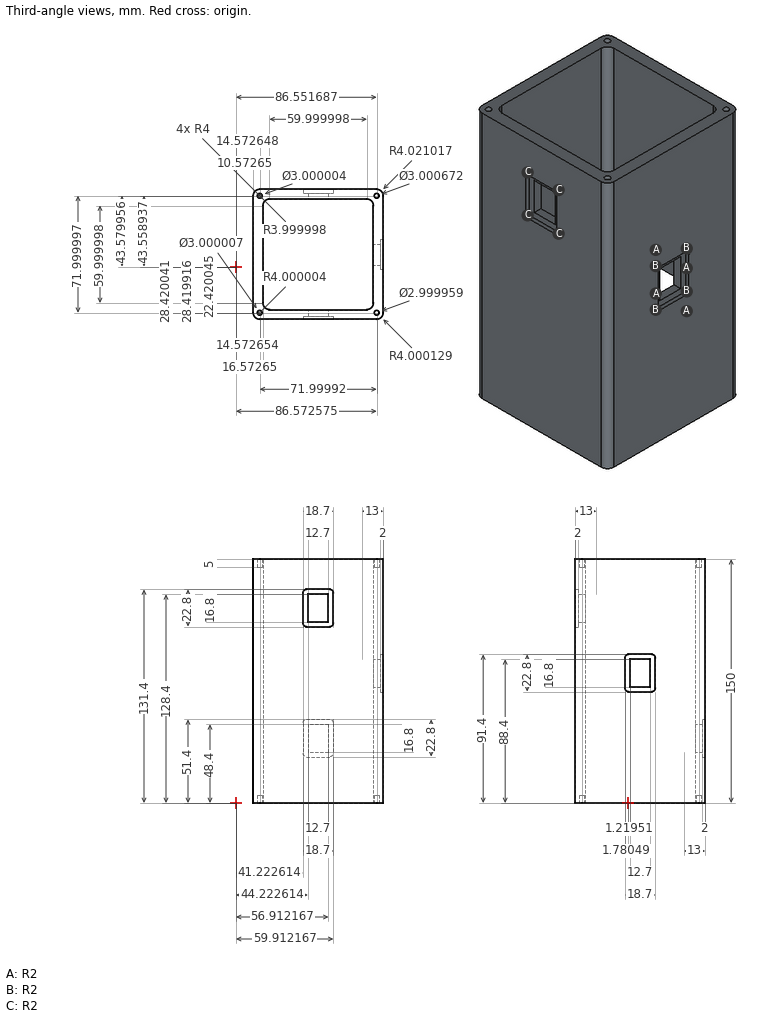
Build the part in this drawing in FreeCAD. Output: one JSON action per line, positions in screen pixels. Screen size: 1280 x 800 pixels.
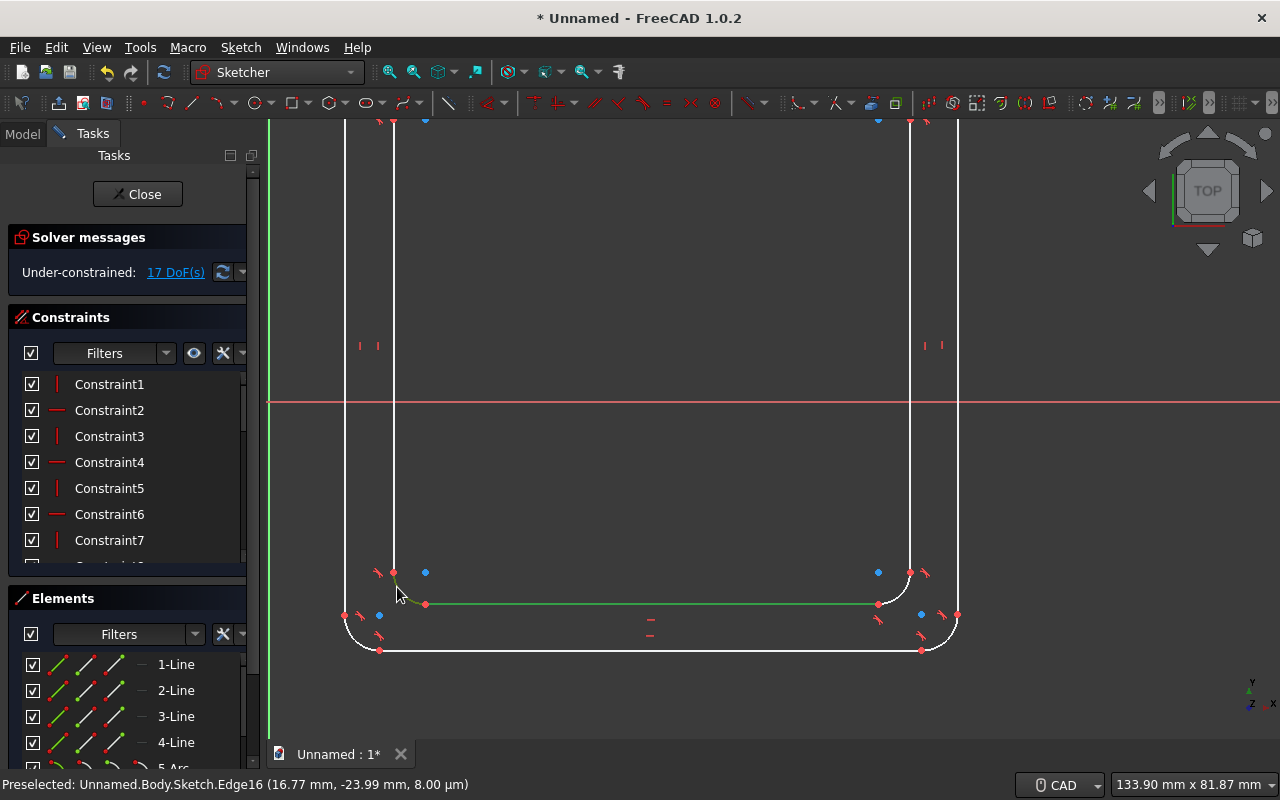
{"action": "left_click", "coordinate": [644, 104]}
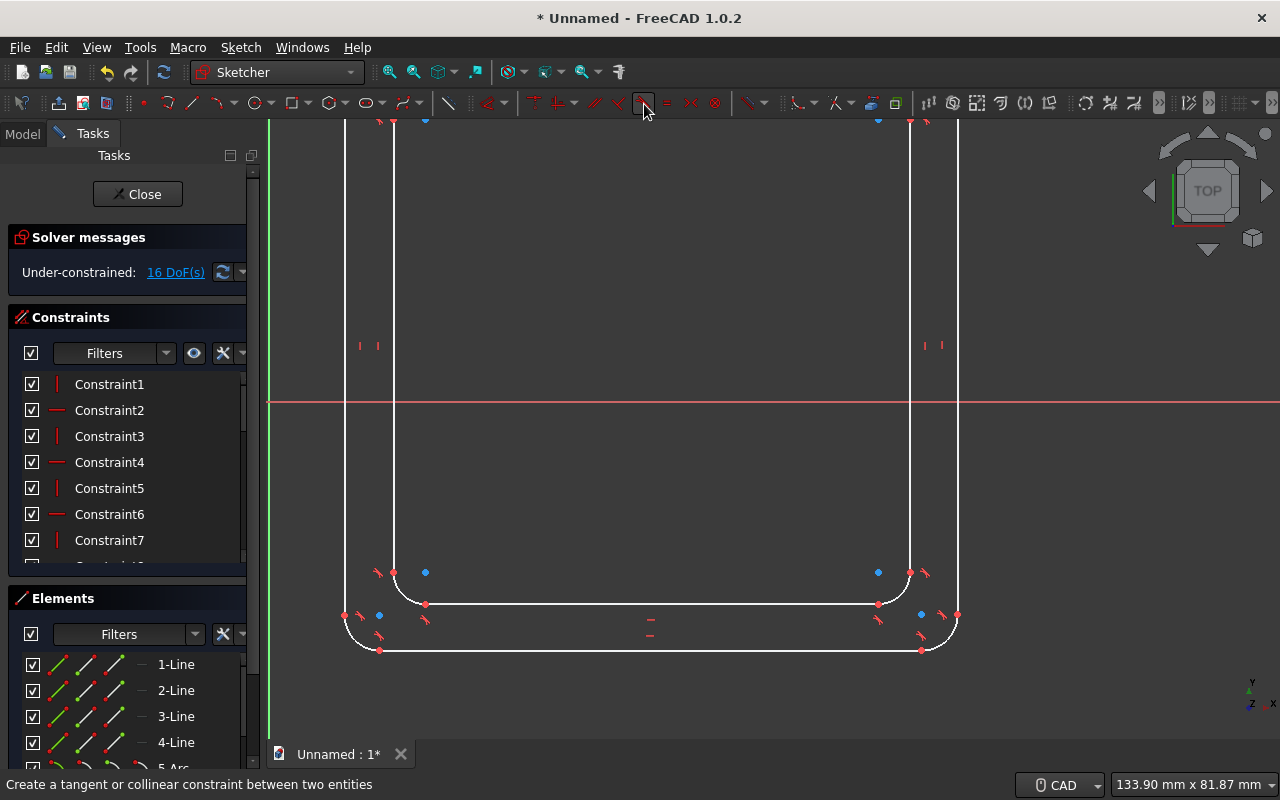
{"action": "scroll", "coordinate": [893, 601], "scroll_direction": "down", "scroll_amount": 2}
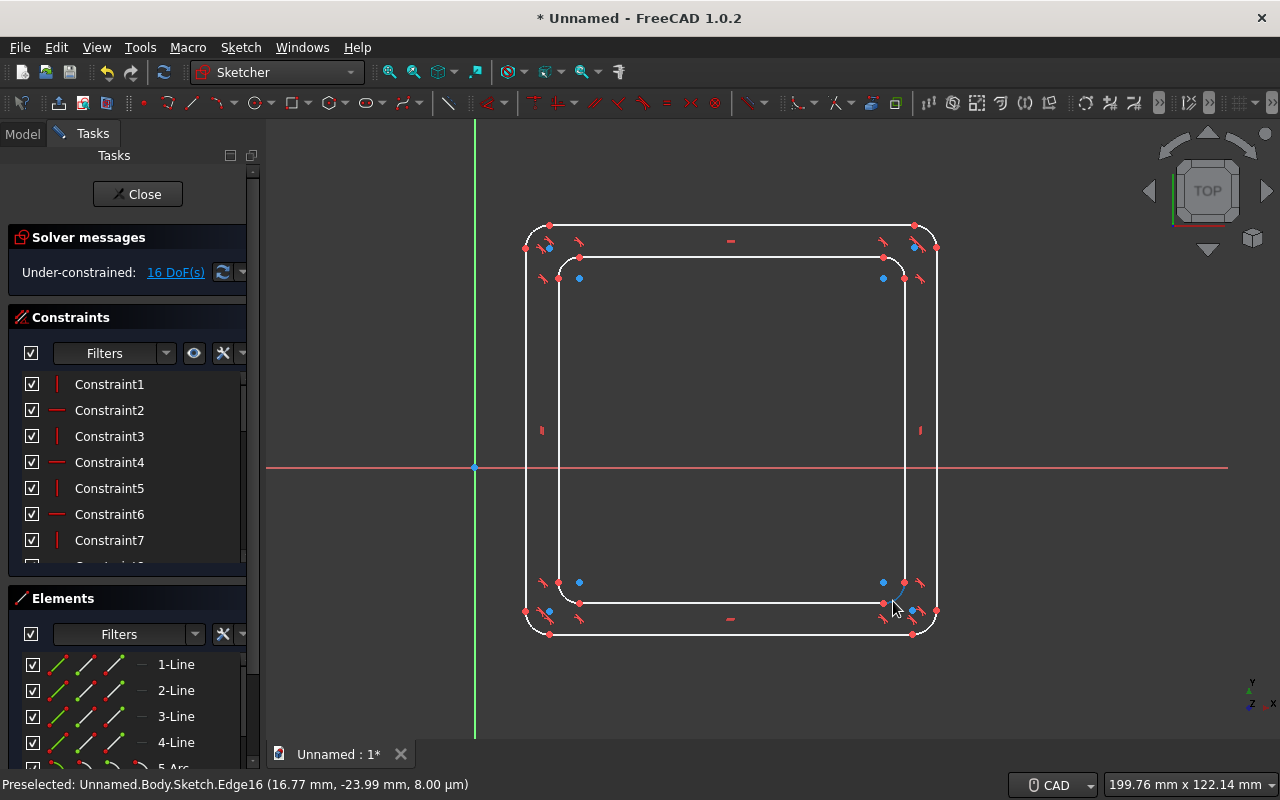
{"action": "scroll", "coordinate": [570, 260], "scroll_direction": "up", "scroll_amount": 2}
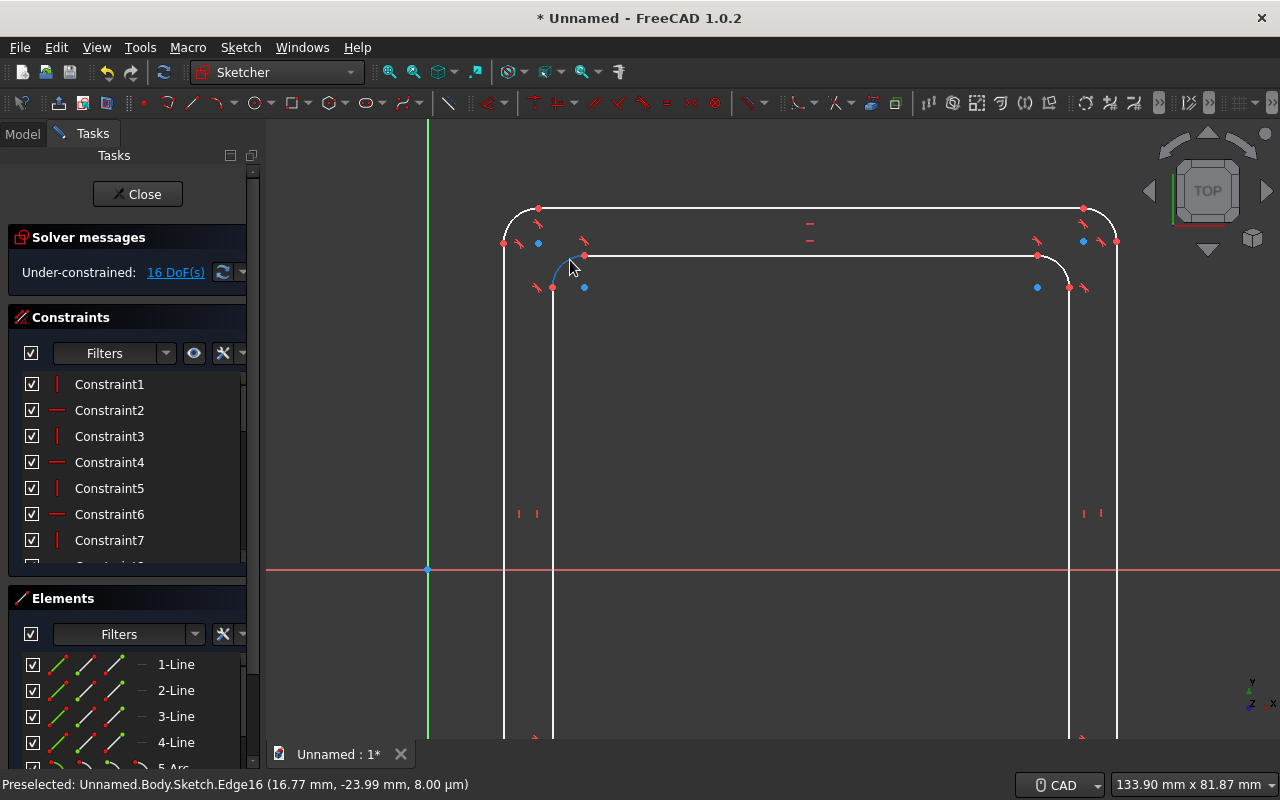
{"action": "left_click", "coordinate": [570, 259]}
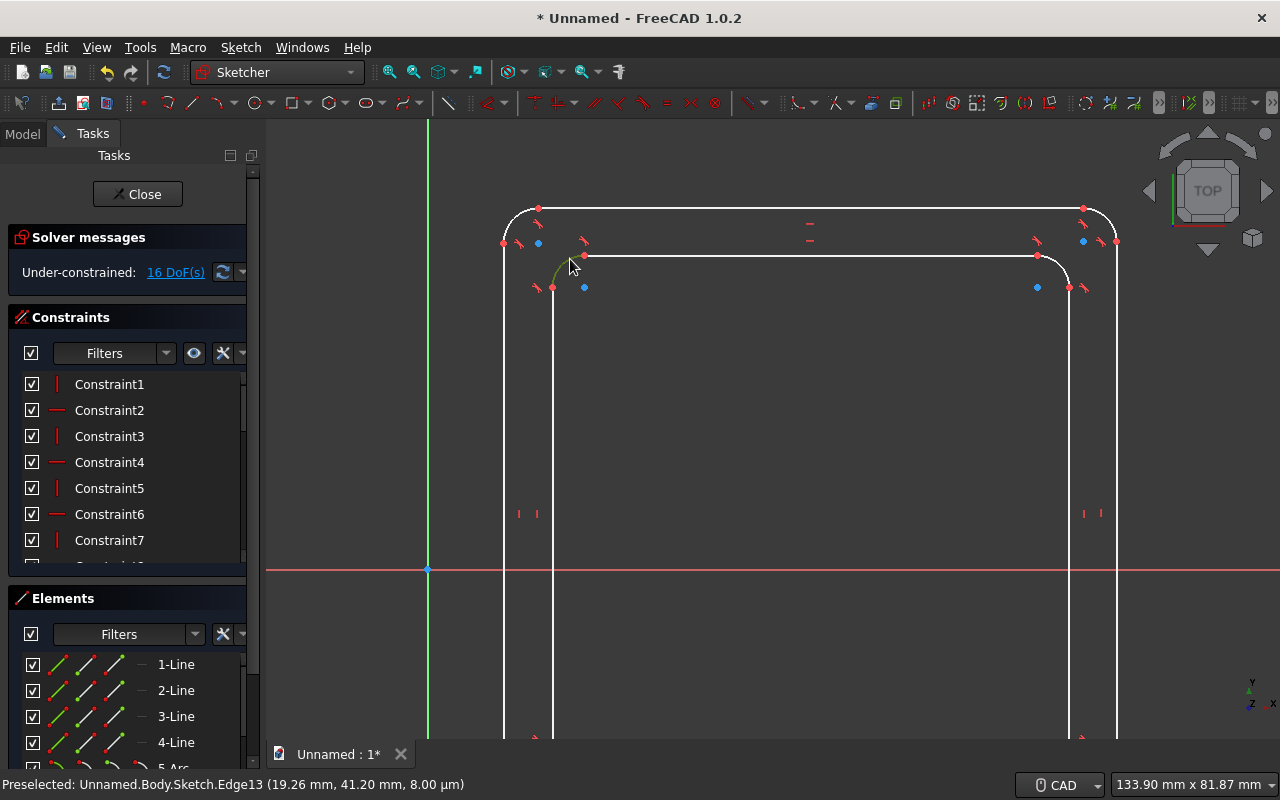
{"action": "left_click", "coordinate": [1066, 273]}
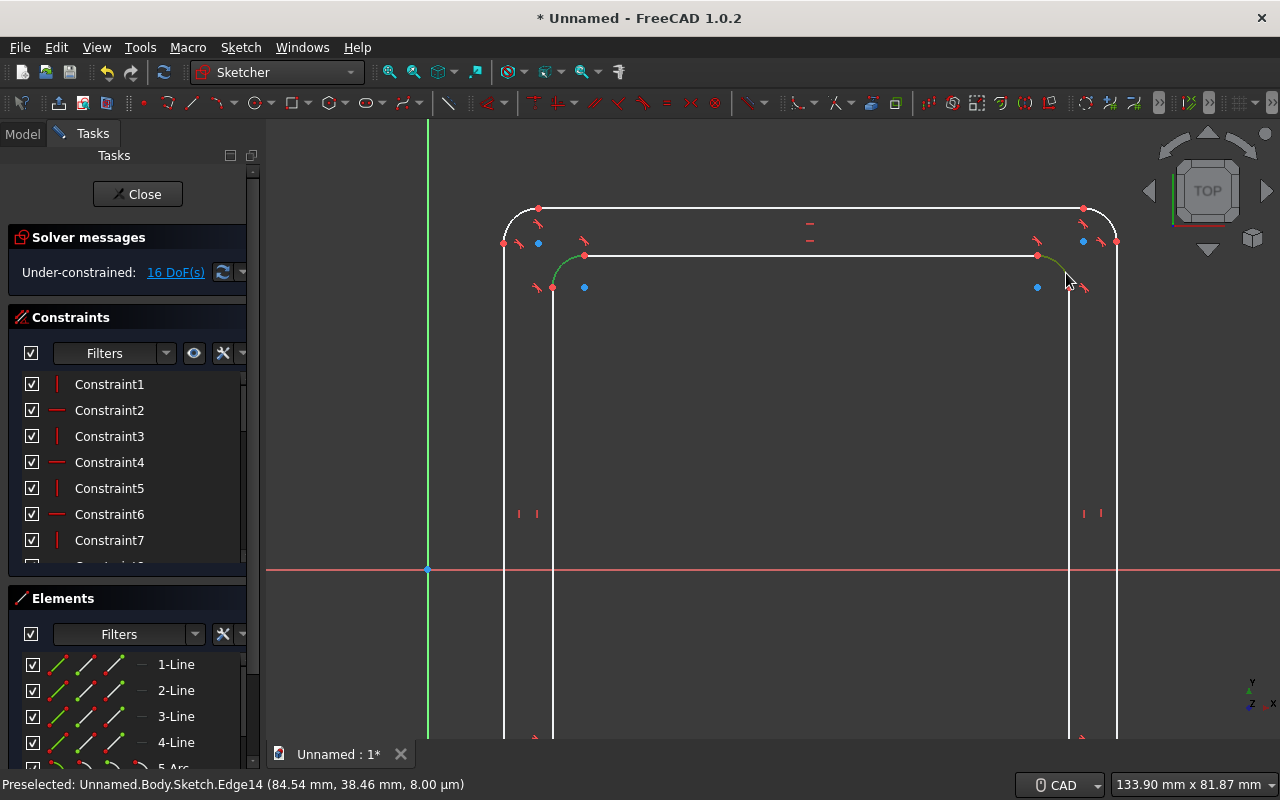
{"action": "scroll", "coordinate": [570, 260], "scroll_direction": "down", "scroll_amount": 2}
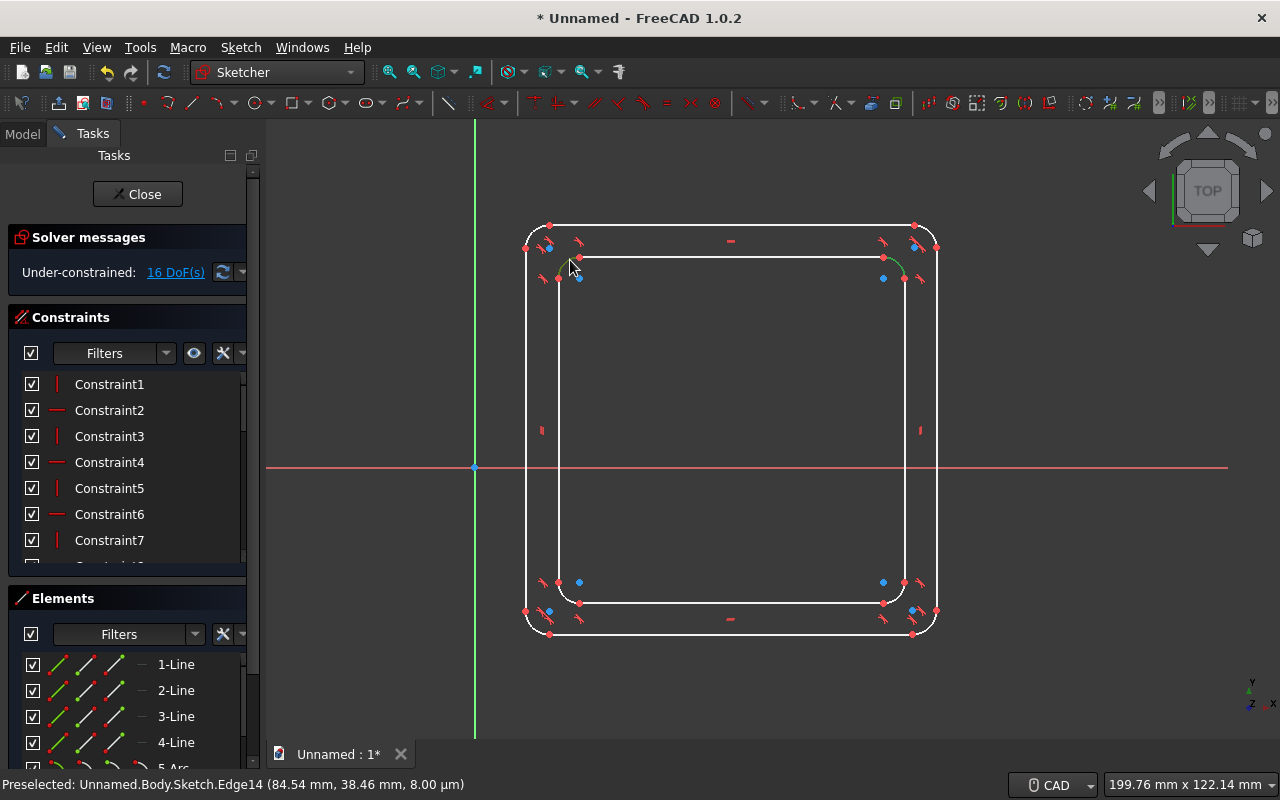
{"action": "scroll", "coordinate": [893, 601], "scroll_direction": "up", "scroll_amount": 2}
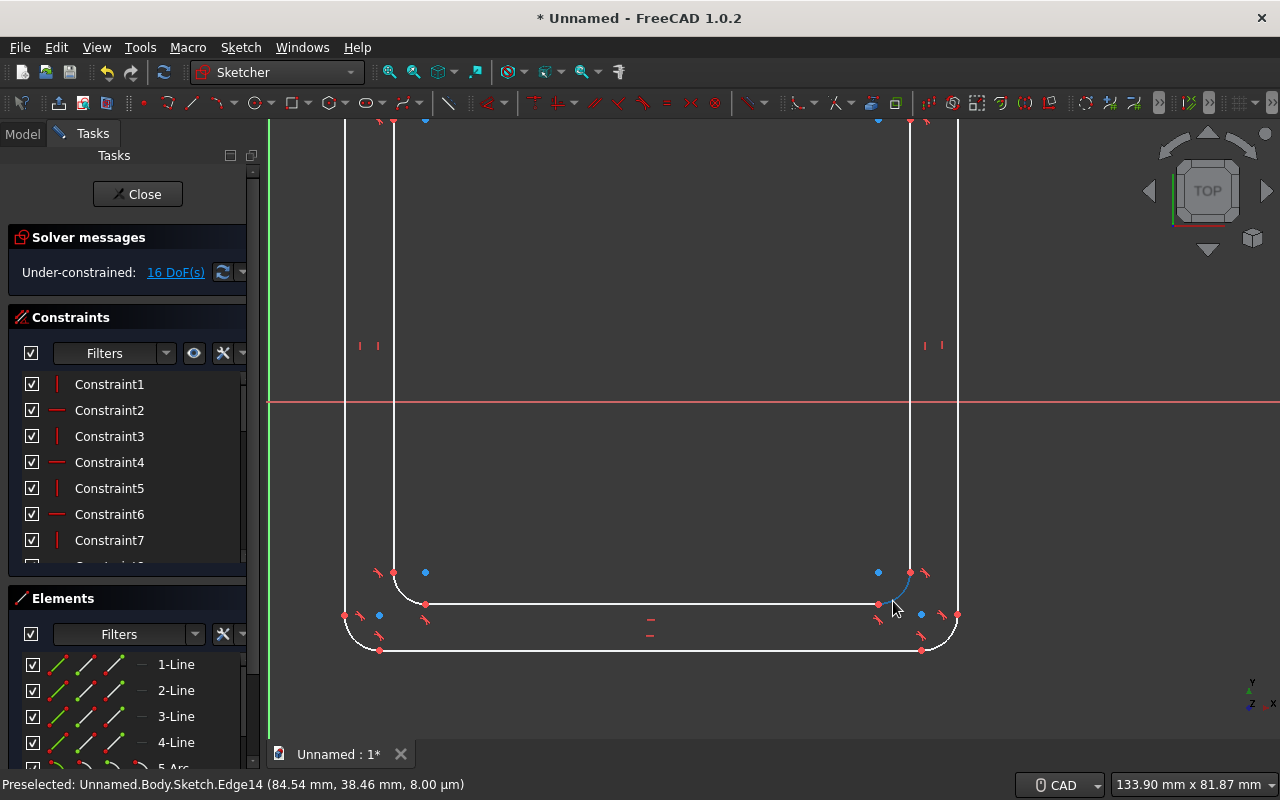
{"action": "left_click", "coordinate": [893, 601]}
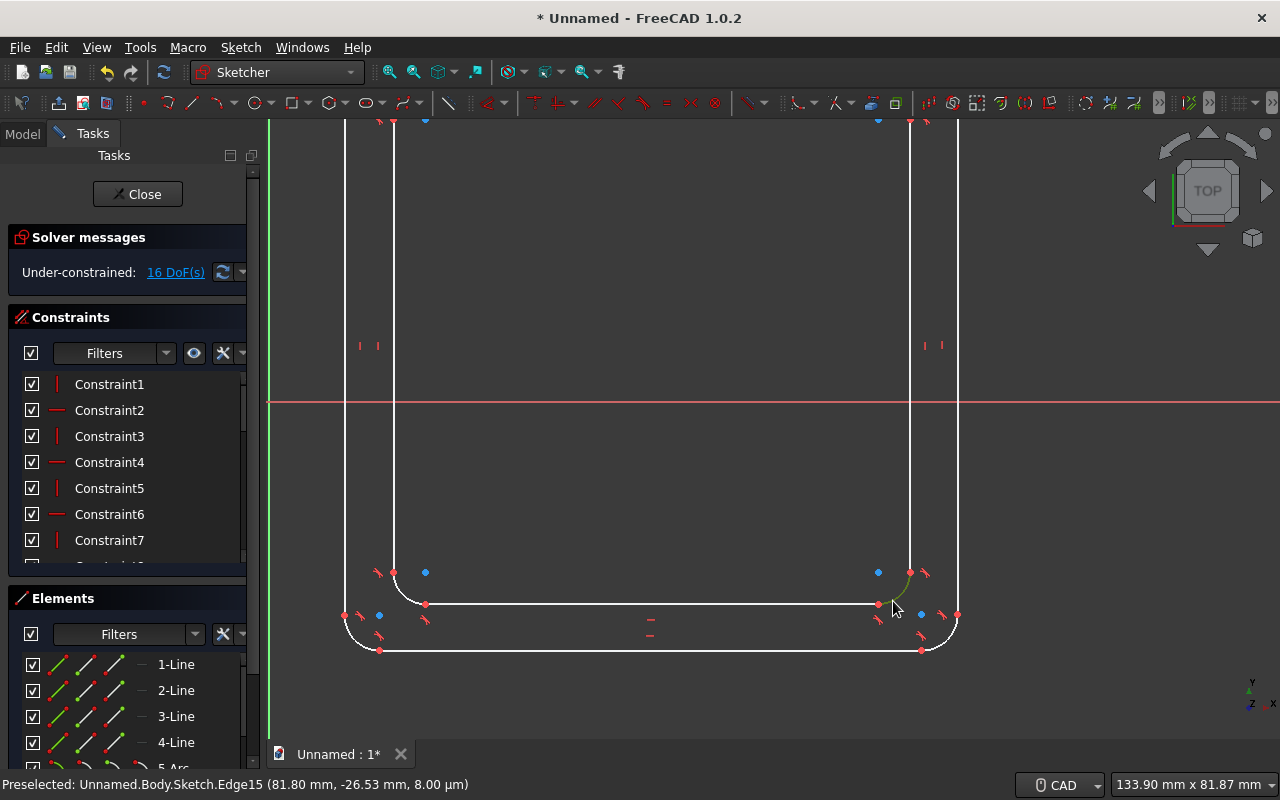
{"action": "left_click", "coordinate": [397, 587]}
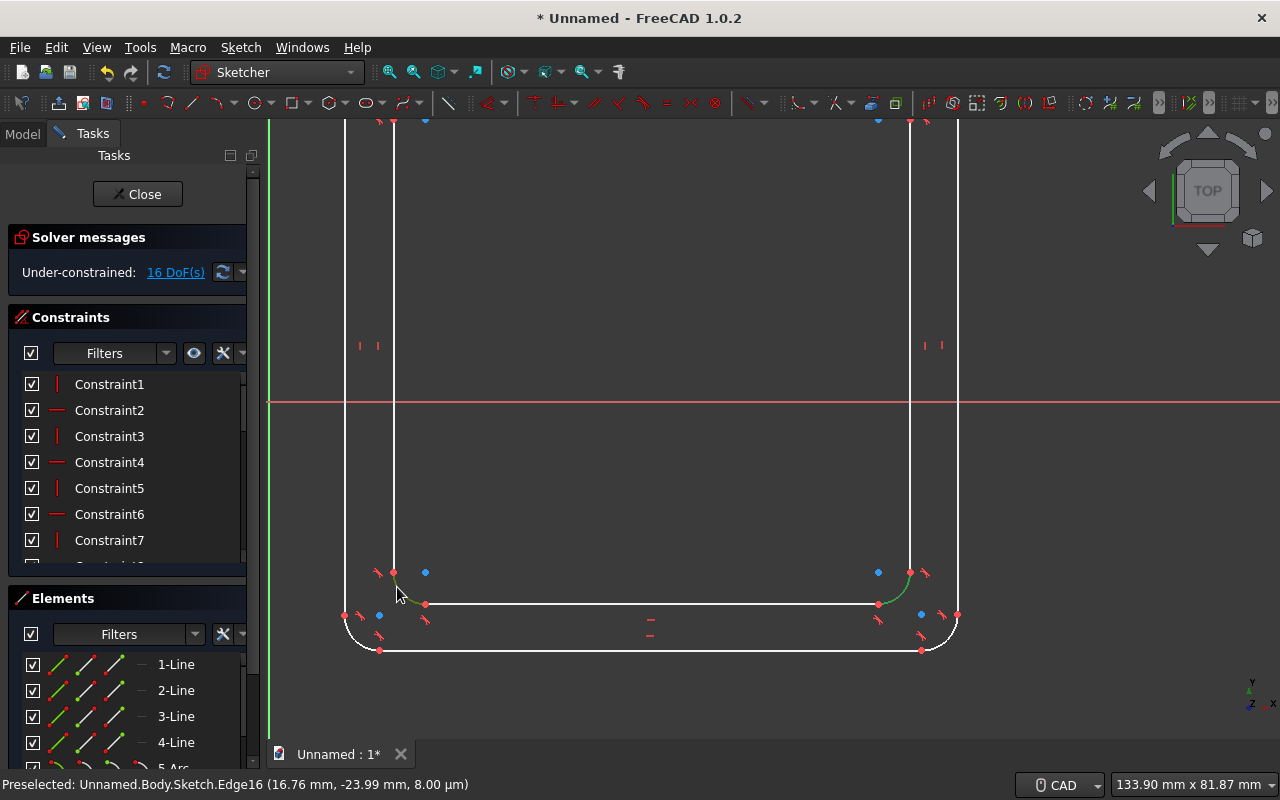
{"action": "left_click", "coordinate": [668, 104]}